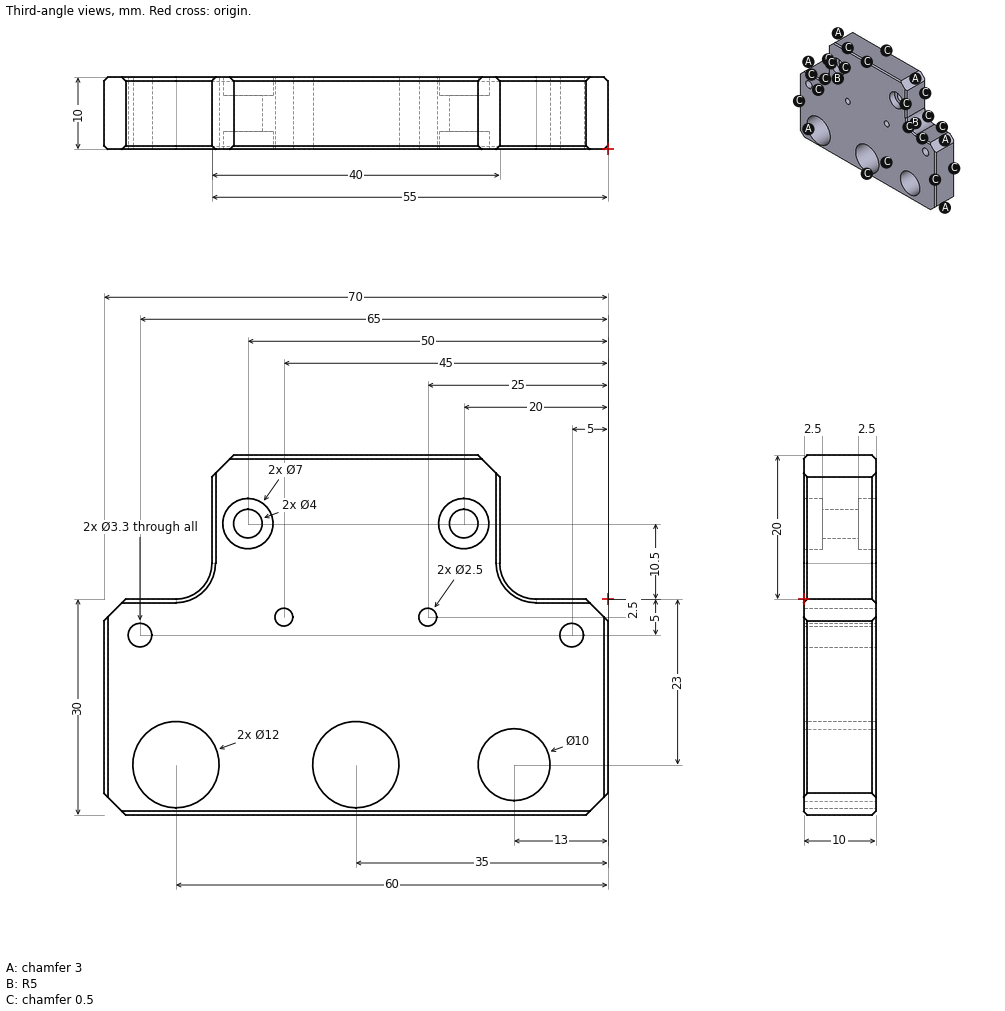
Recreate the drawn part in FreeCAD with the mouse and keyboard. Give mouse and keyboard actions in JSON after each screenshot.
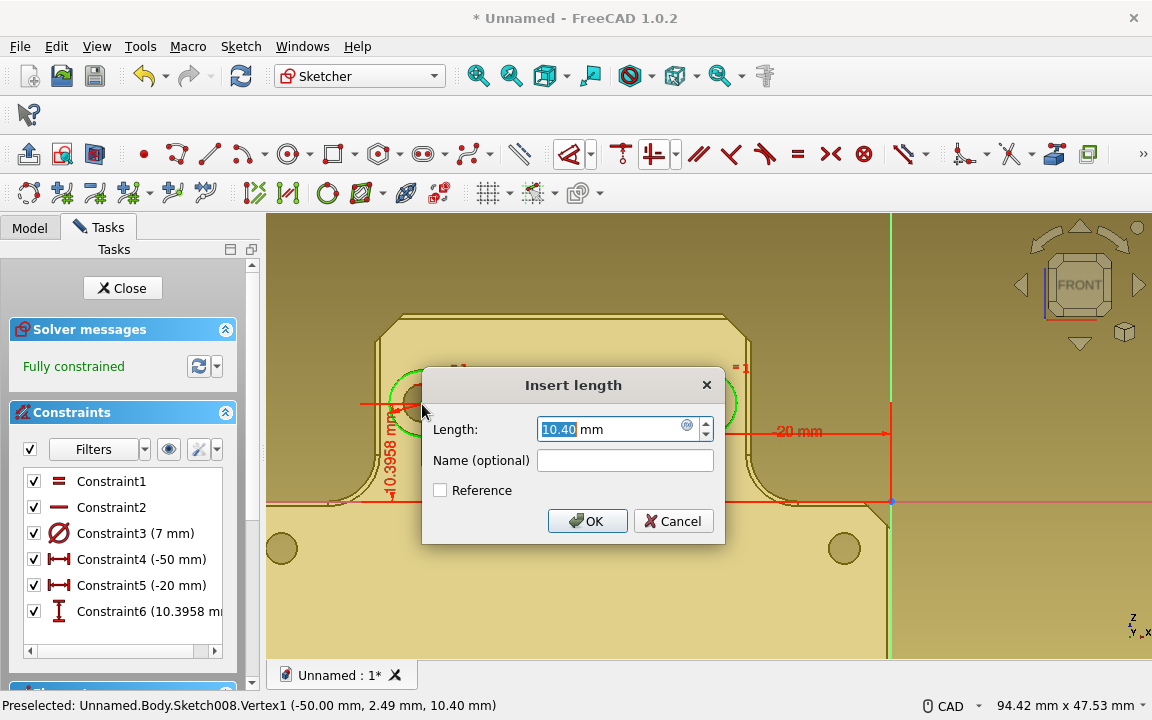
{"action": "type", "text": "10.5"}
{"action": "key", "text": "Return"}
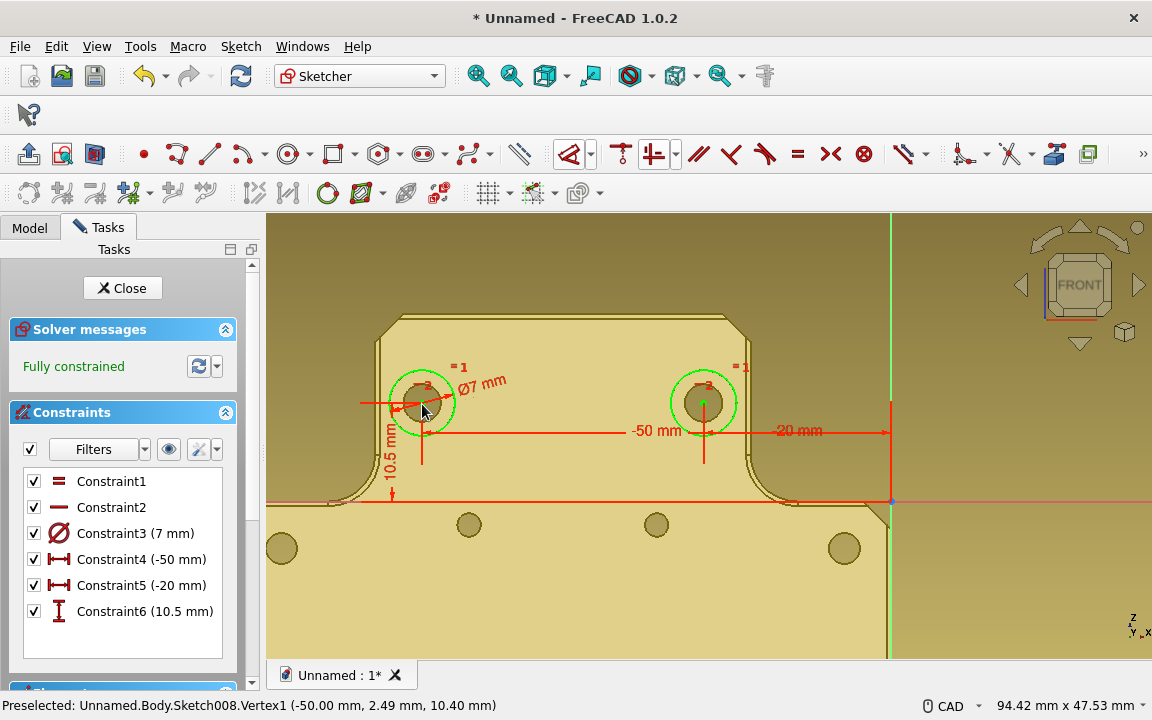
{"action": "left_click", "coordinate": [123, 288]}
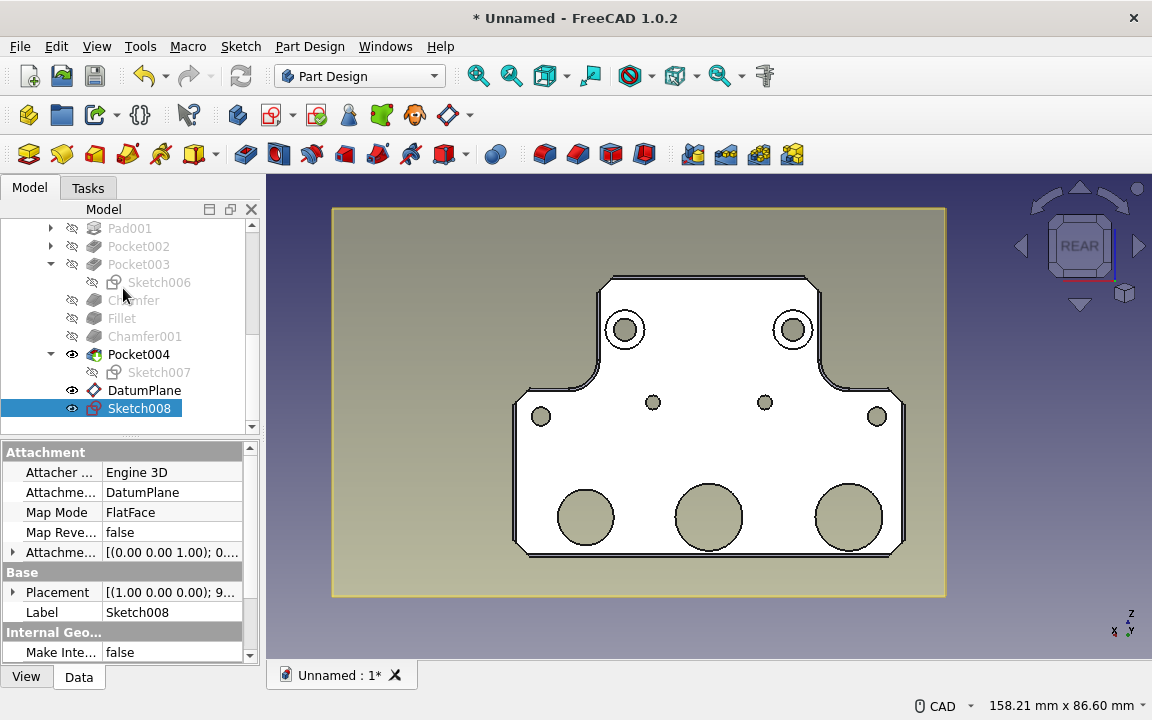
{"action": "left_click", "coordinate": [246, 154]}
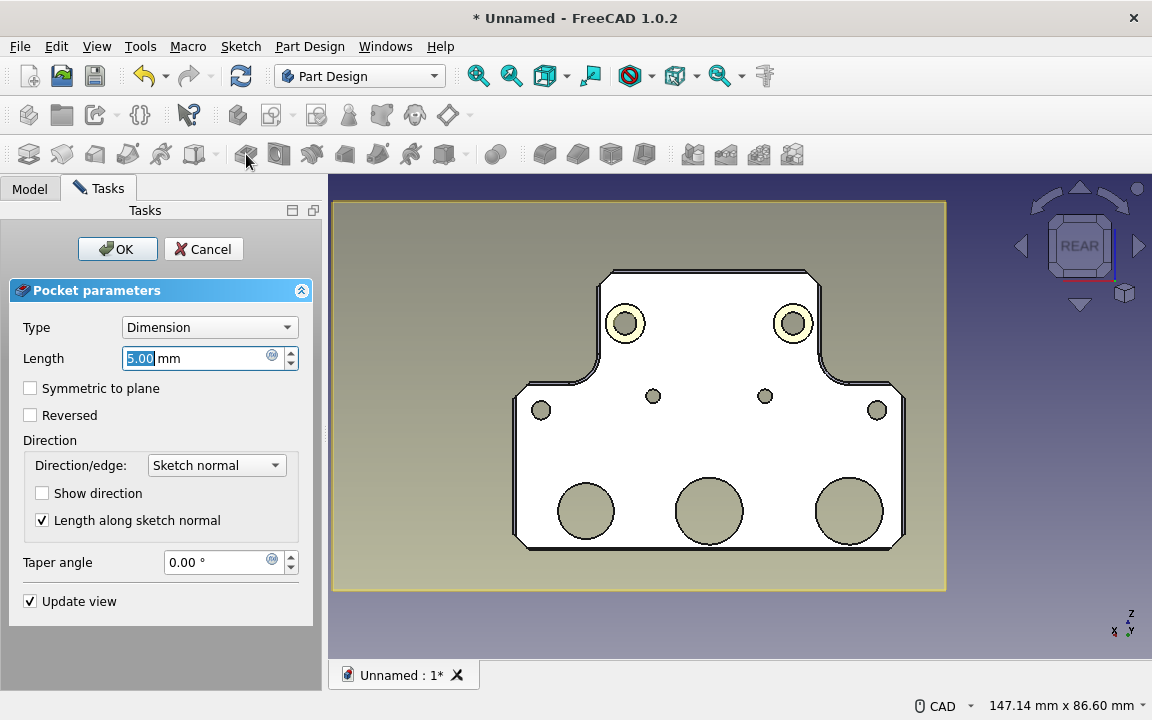
{"action": "type", "text": "2.5"}
{"action": "key", "text": "Tab"}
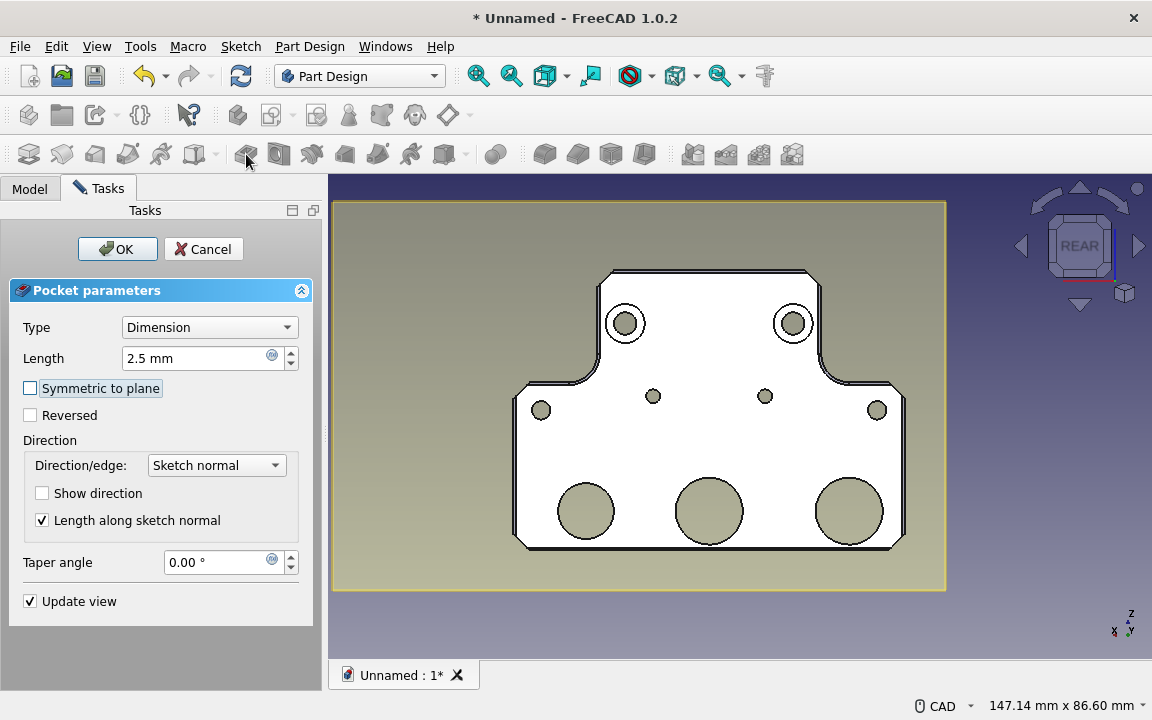
{"action": "left_click", "coordinate": [31, 415]}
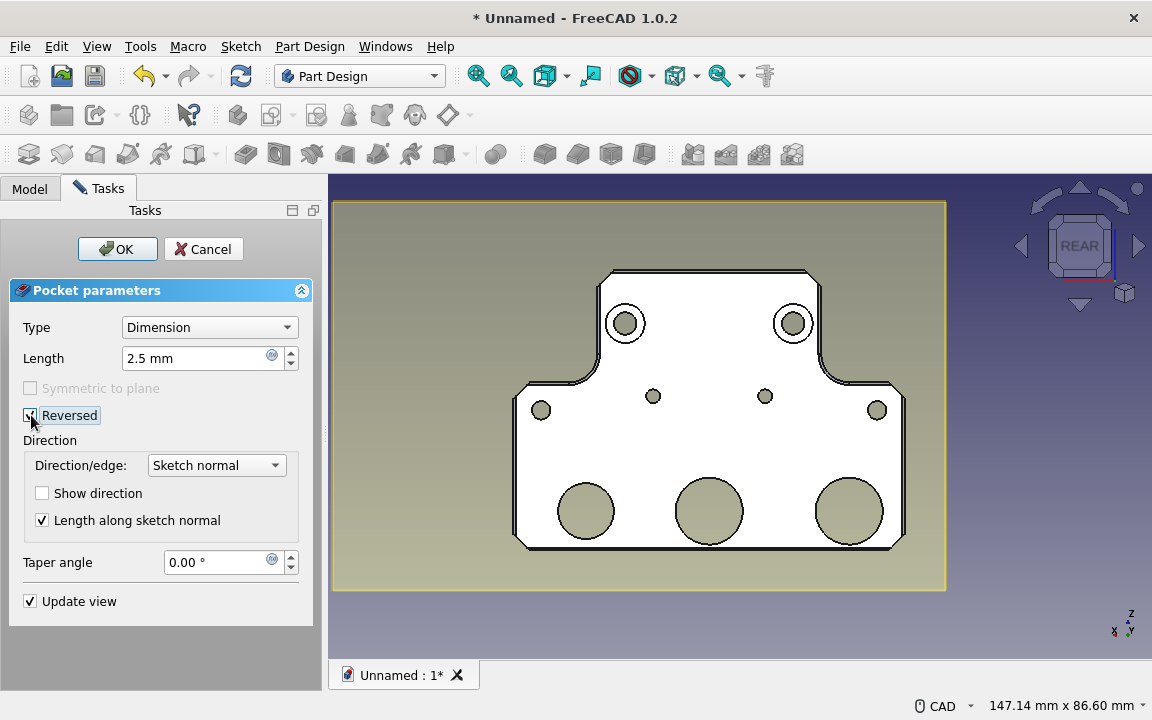
{"action": "left_click", "coordinate": [118, 249]}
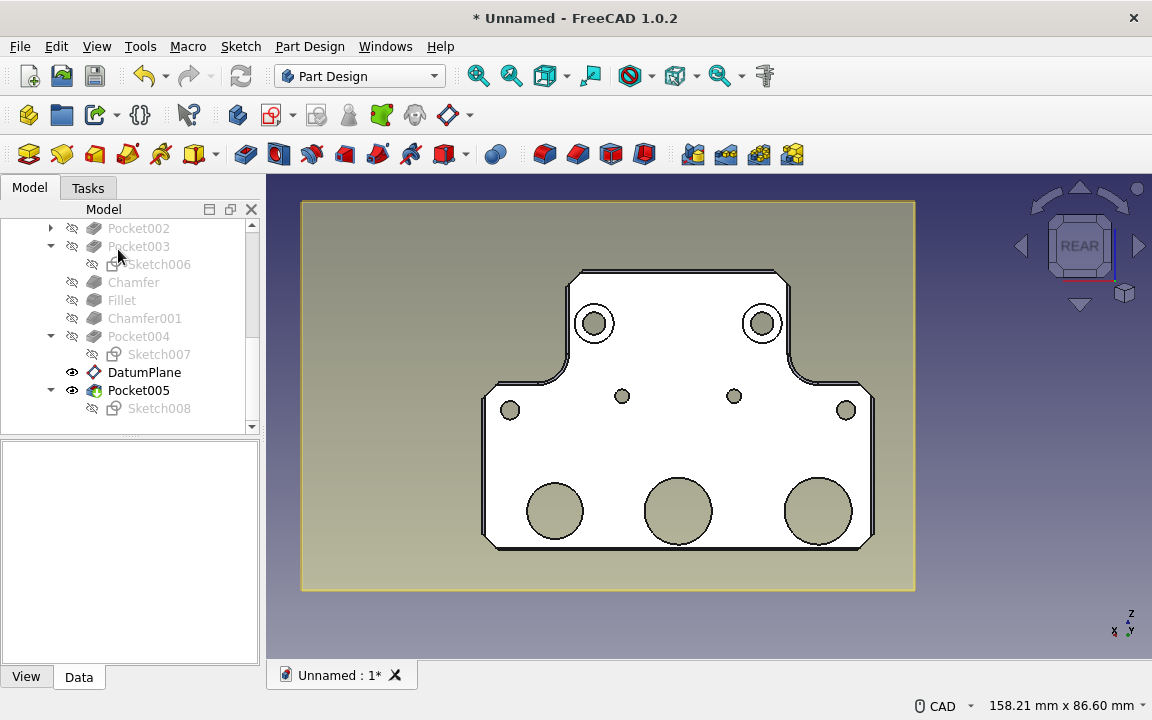
{"action": "left_click", "coordinate": [117, 372]}
{"action": "key", "text": "space"}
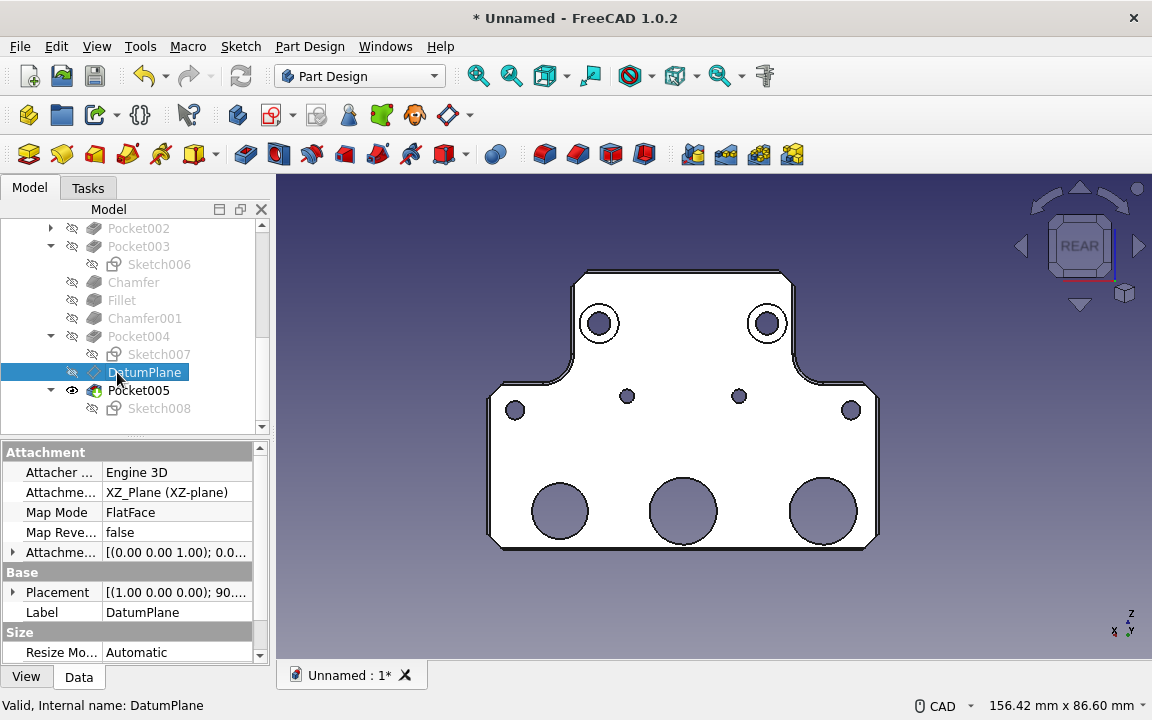
{"action": "key", "text": "0"}